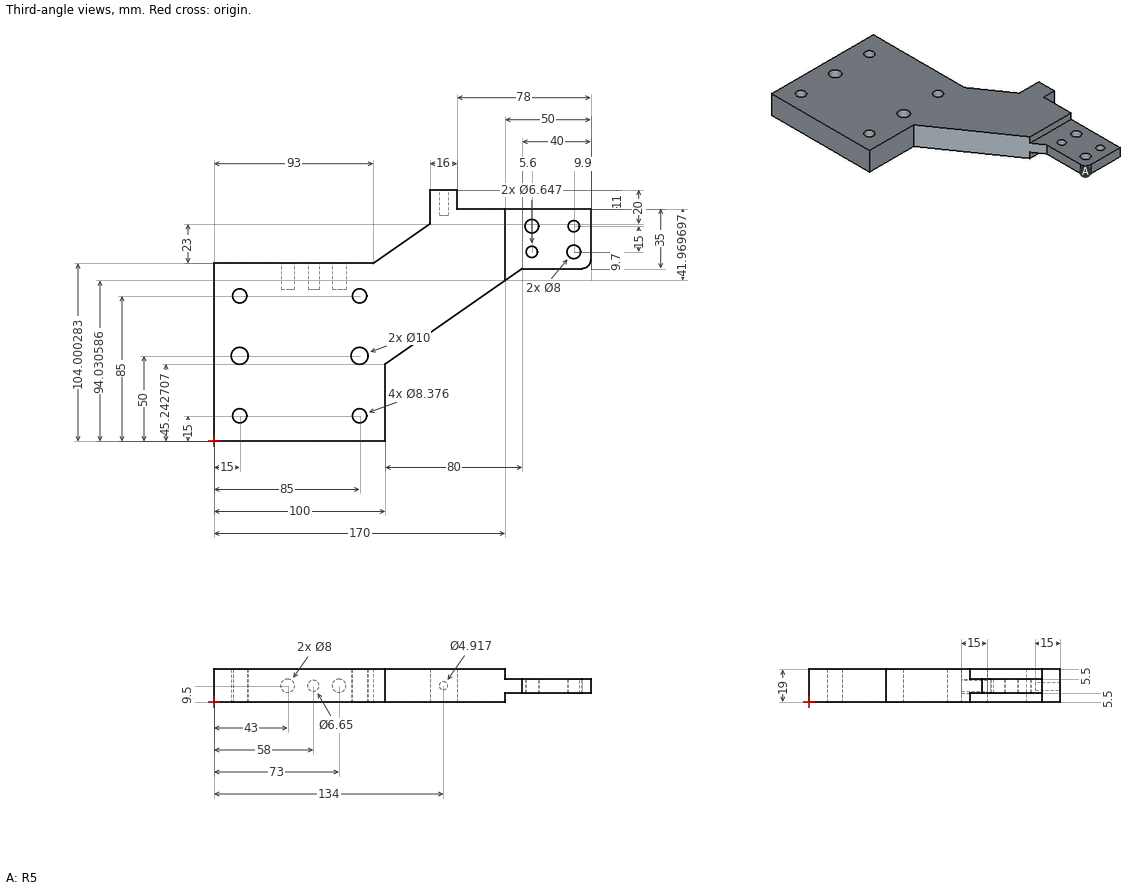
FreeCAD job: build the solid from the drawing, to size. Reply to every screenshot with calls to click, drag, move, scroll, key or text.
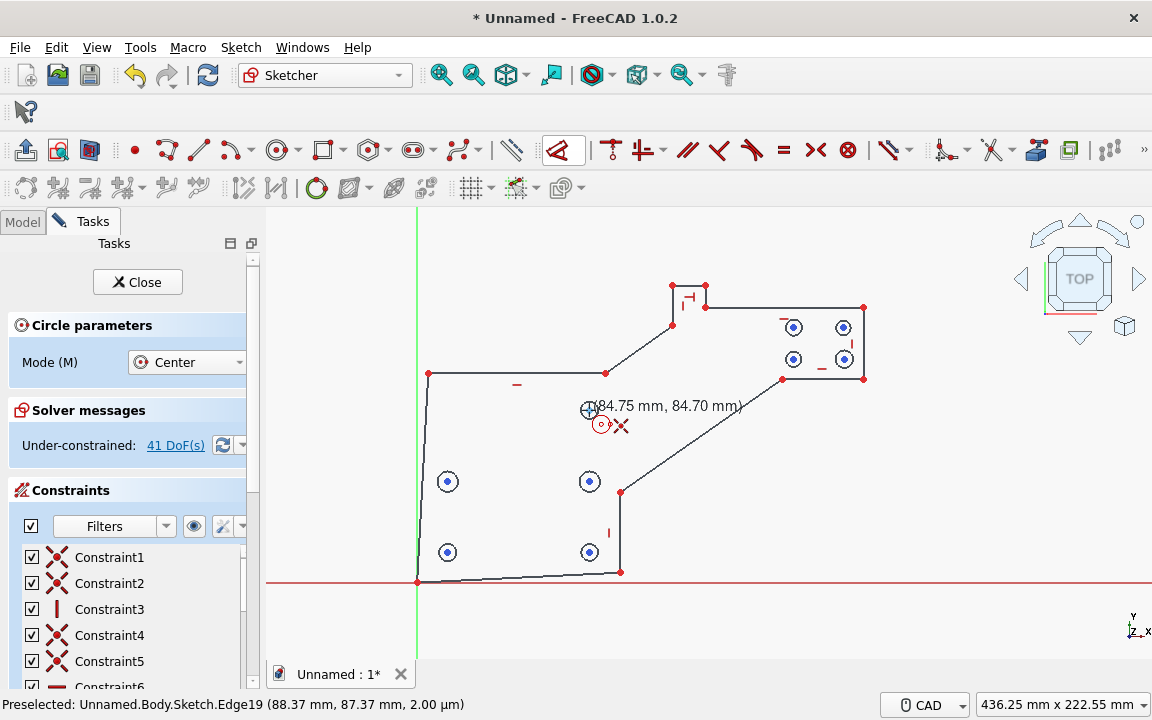
scroll(448, 410, up, 5)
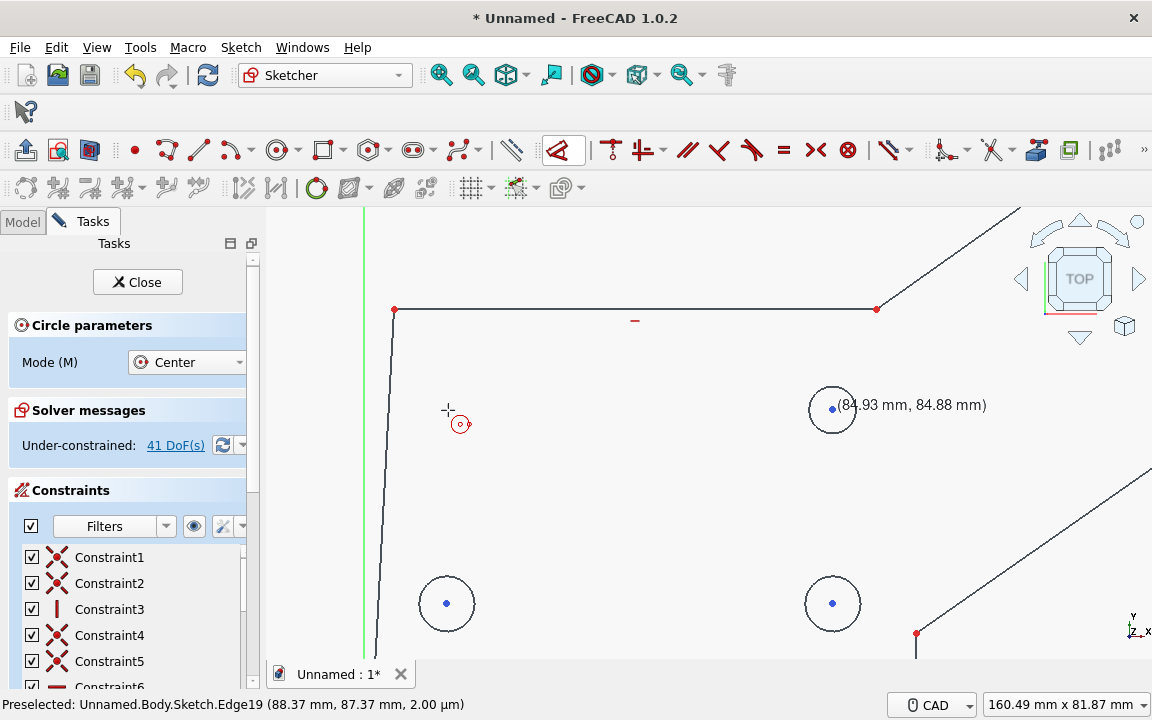
click(446, 409)
click(463, 393)
key(Escape)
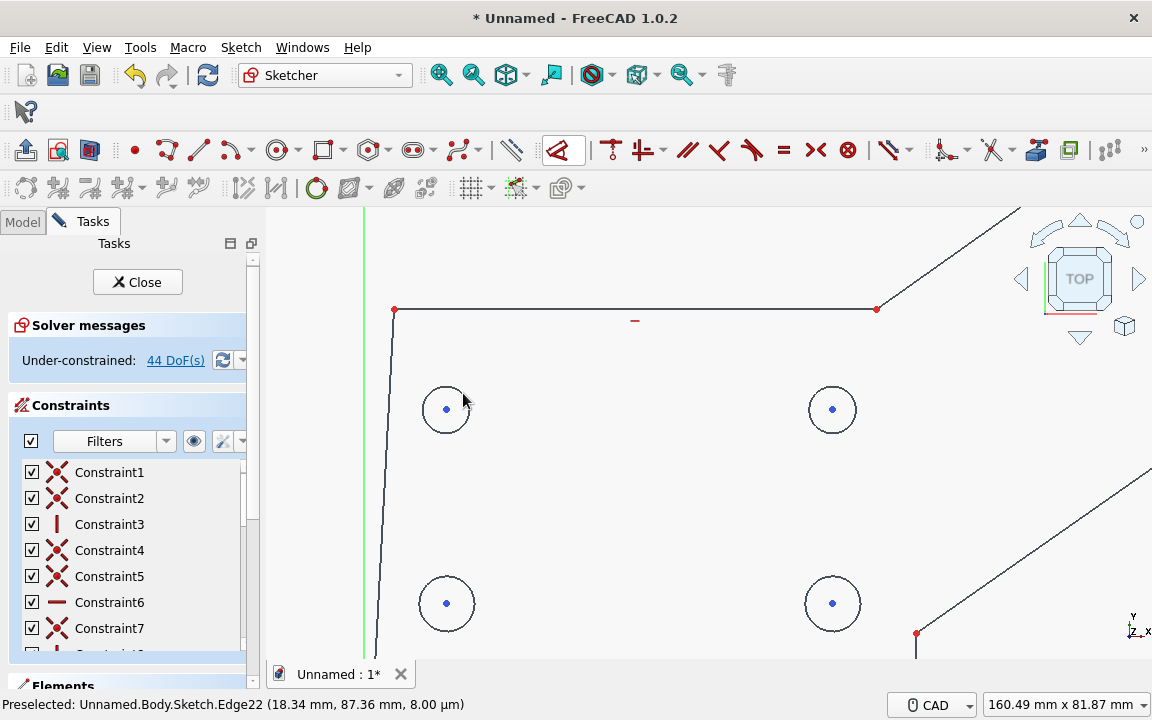
scroll(448, 410, down, 5)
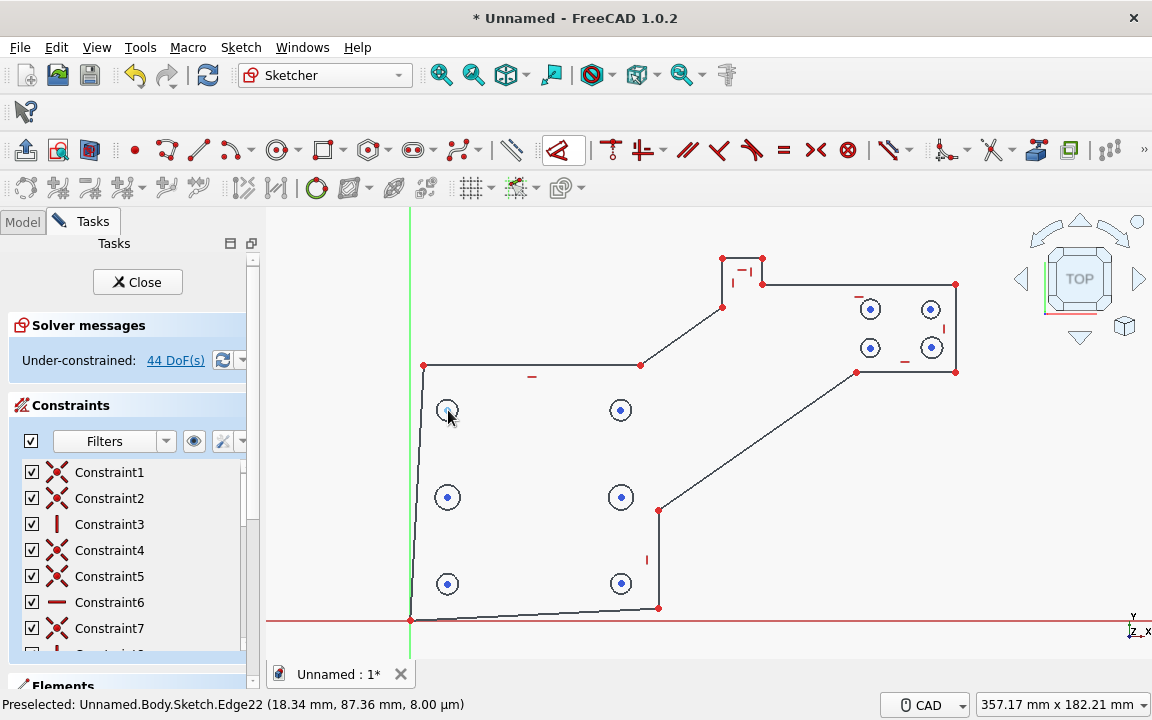
scroll(559, 576, up, 4)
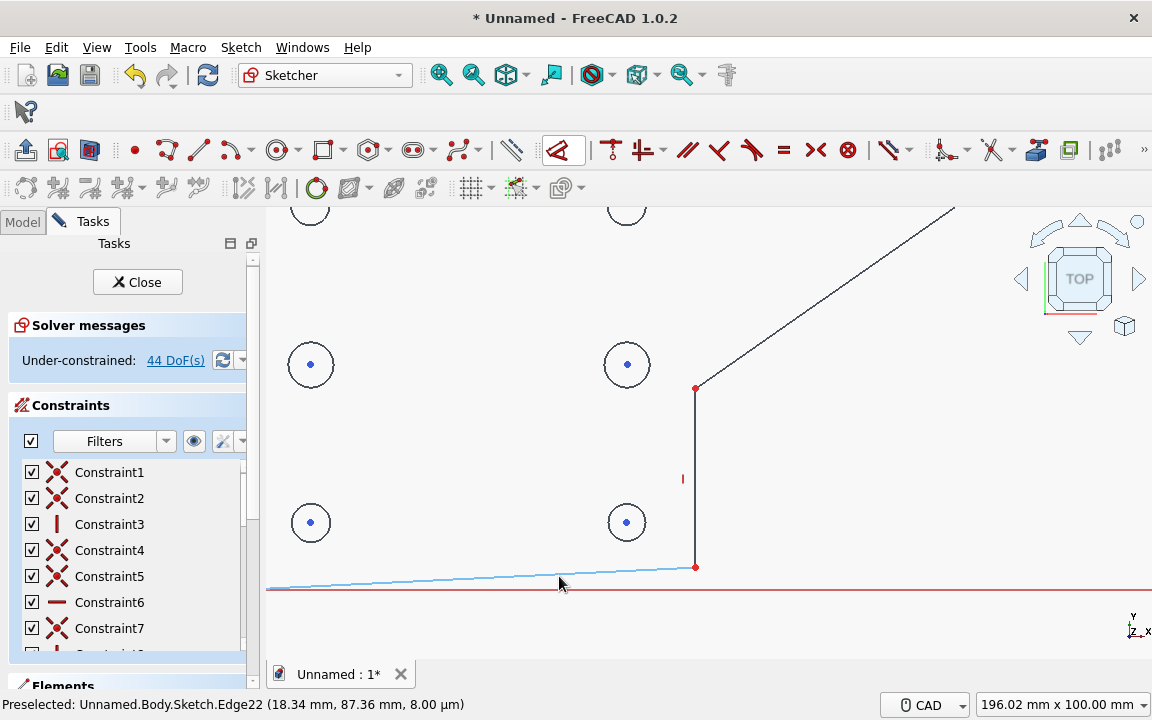
click(560, 574)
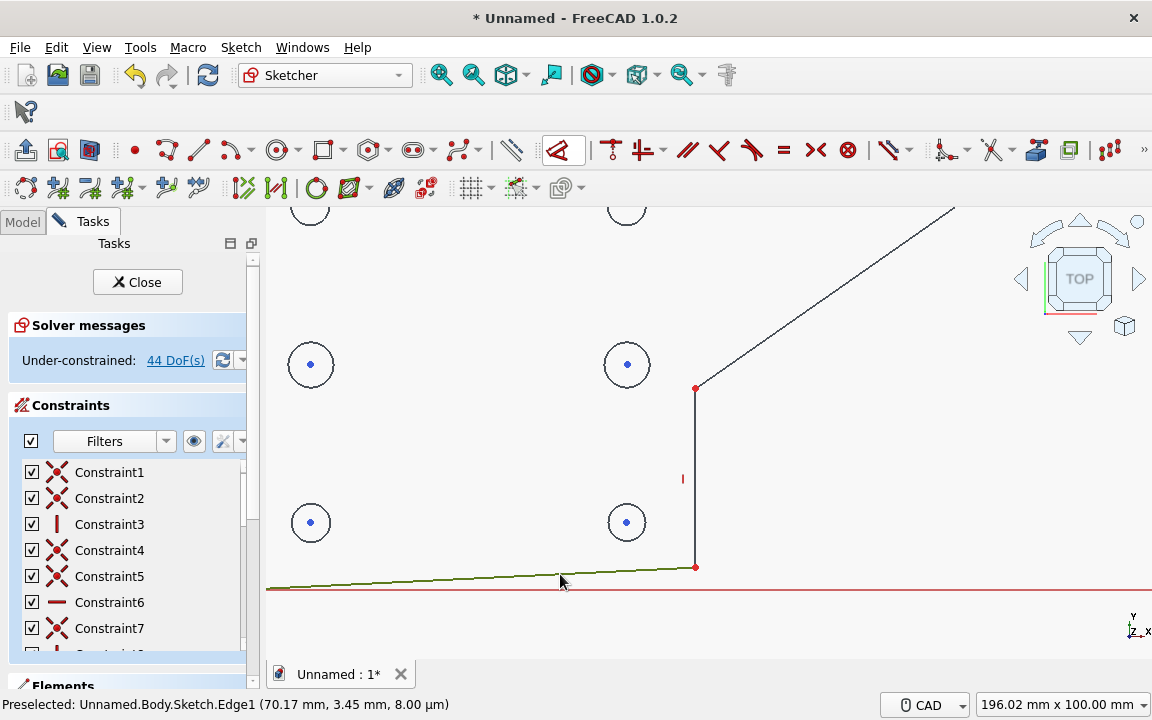
click(666, 150)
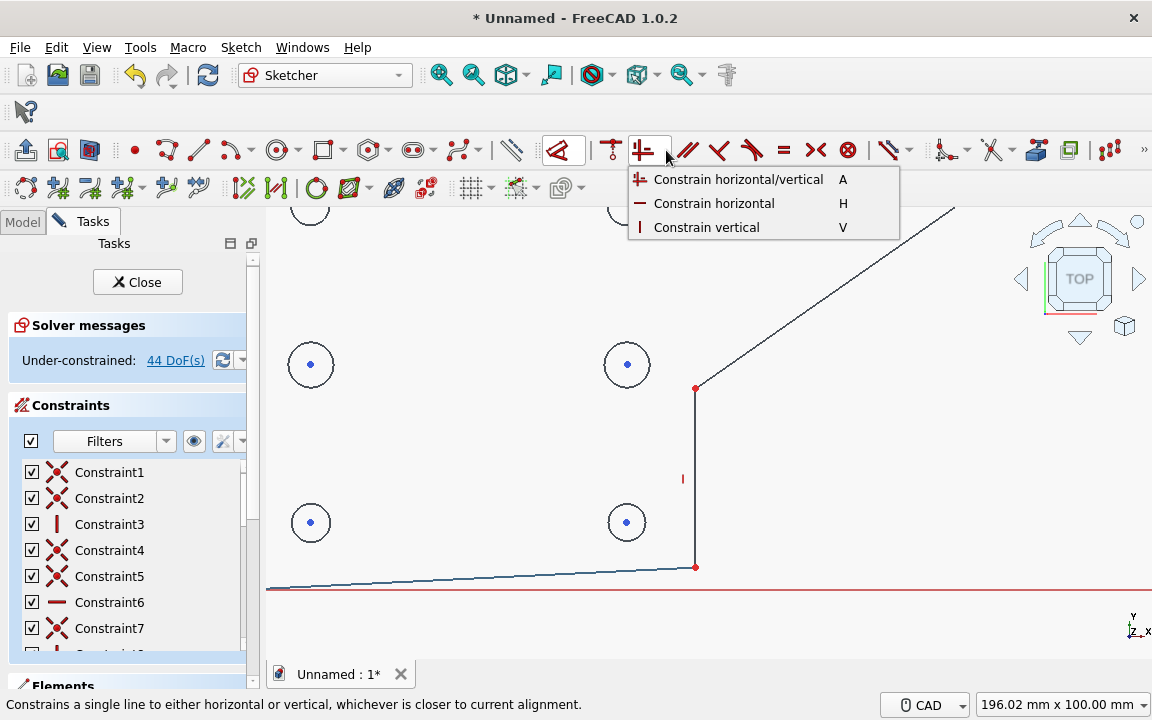
click(764, 203)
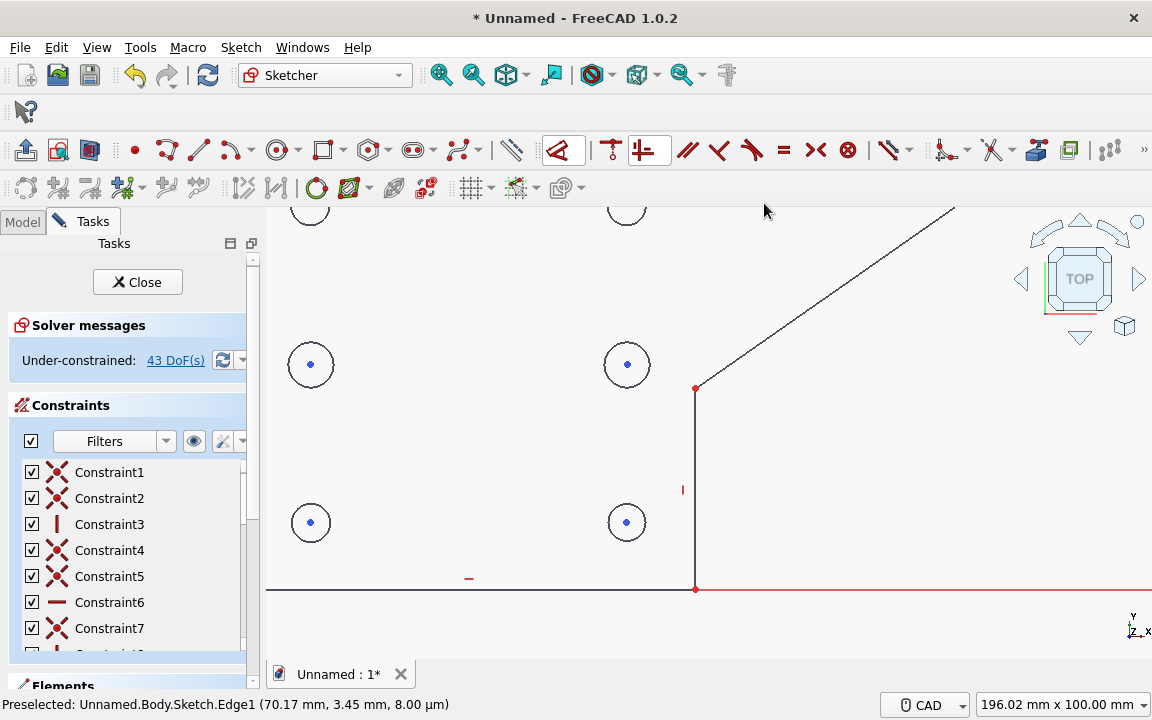
scroll(559, 576, down, 4)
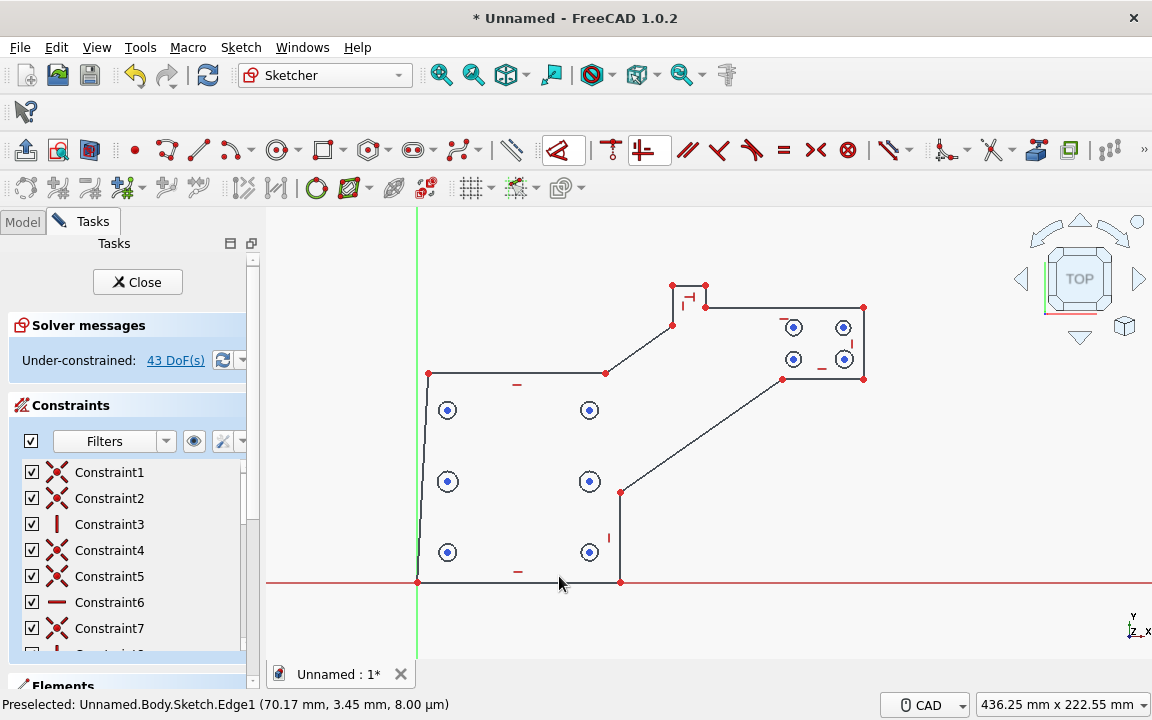
scroll(425, 436, up, 3)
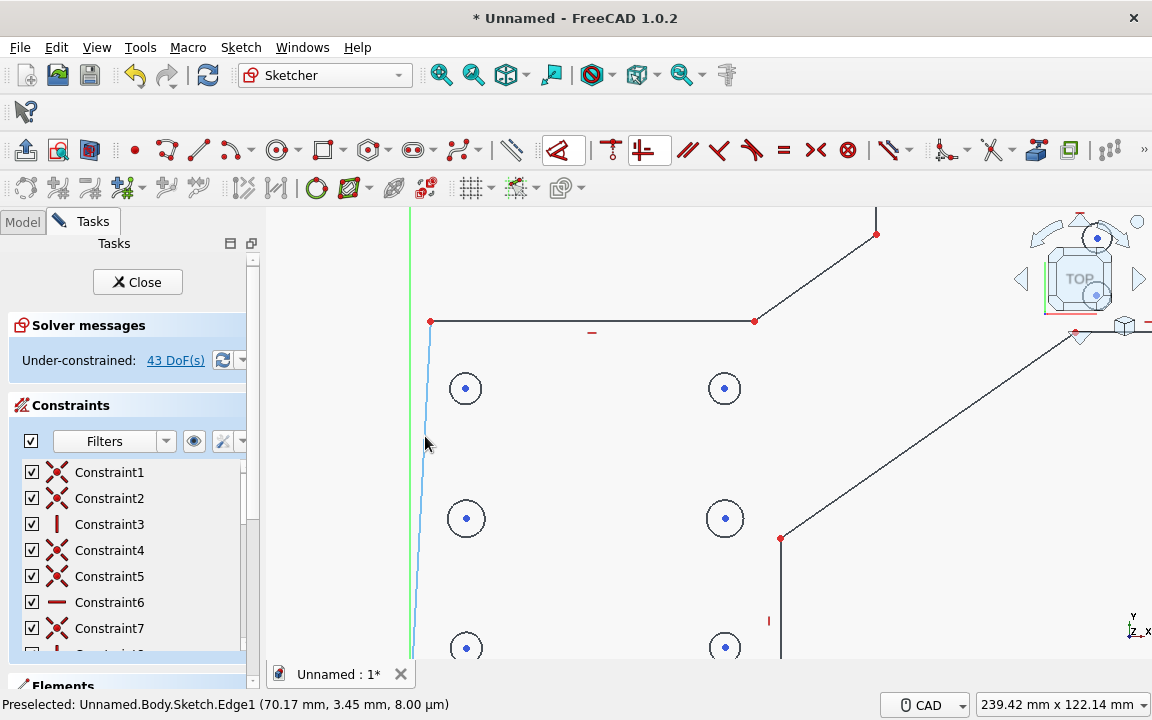
click(425, 436)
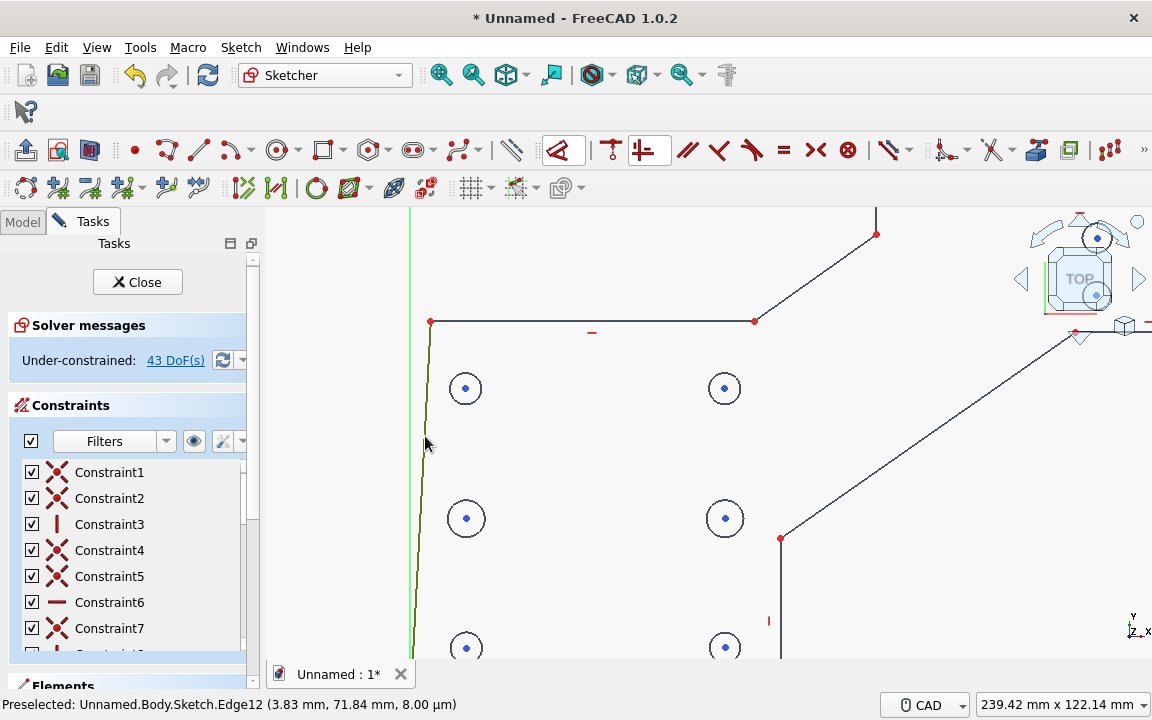
click(666, 150)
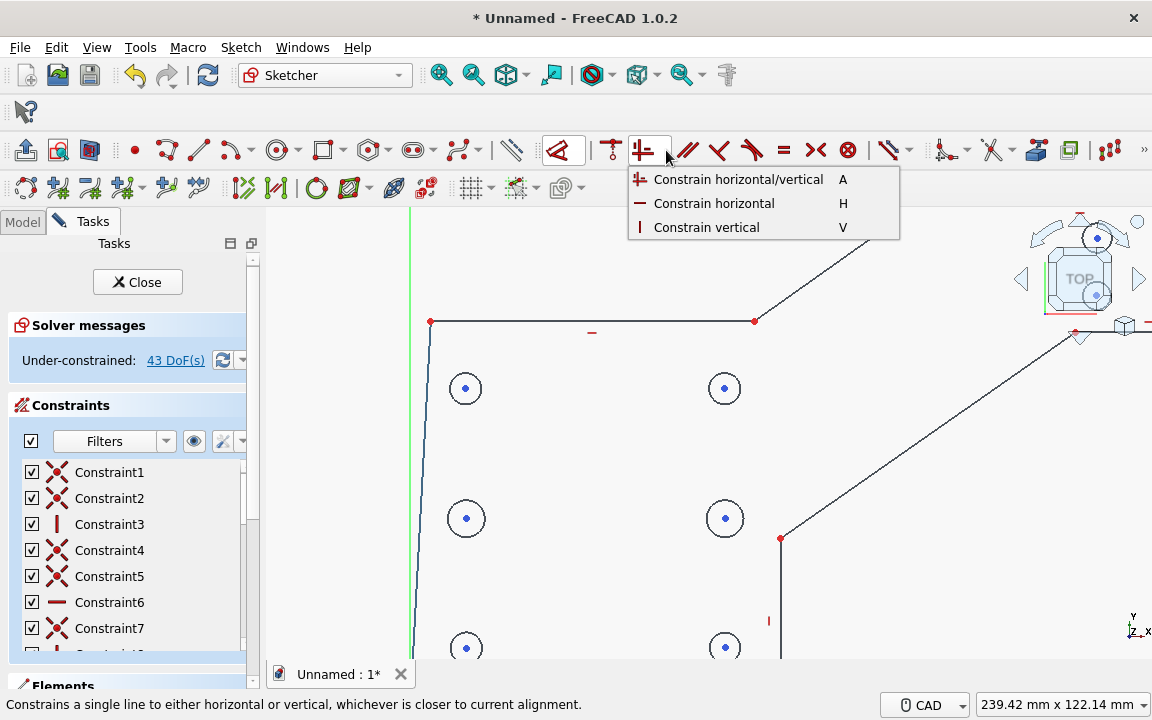
click(764, 227)